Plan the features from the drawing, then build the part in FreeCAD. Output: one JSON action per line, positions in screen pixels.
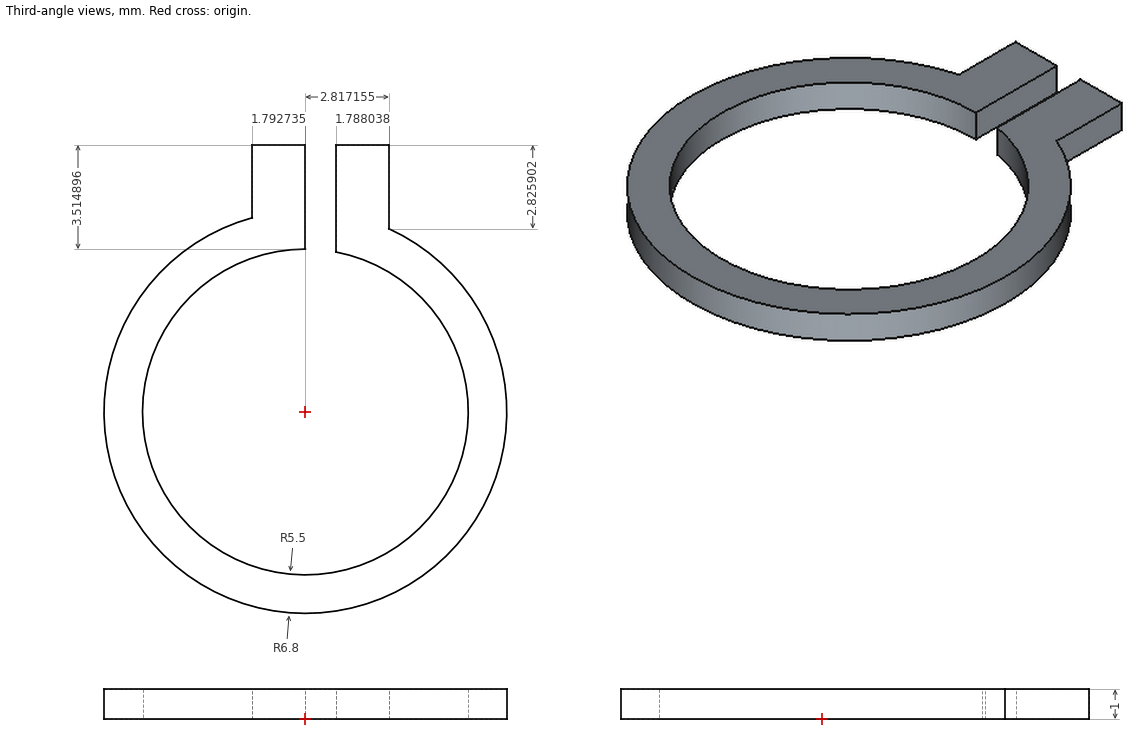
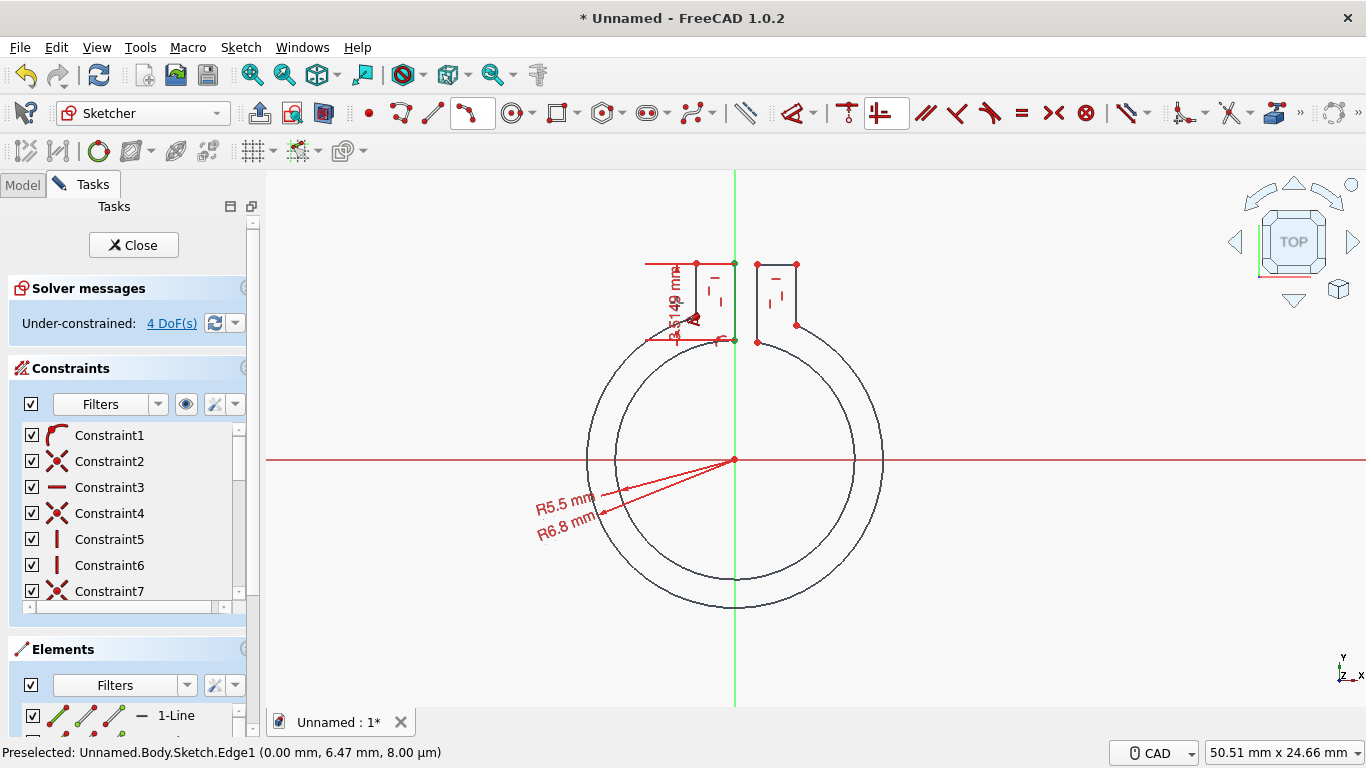
{"action": "left_click", "coordinate": [723, 264]}
{"action": "left_click", "coordinate": [715, 230]}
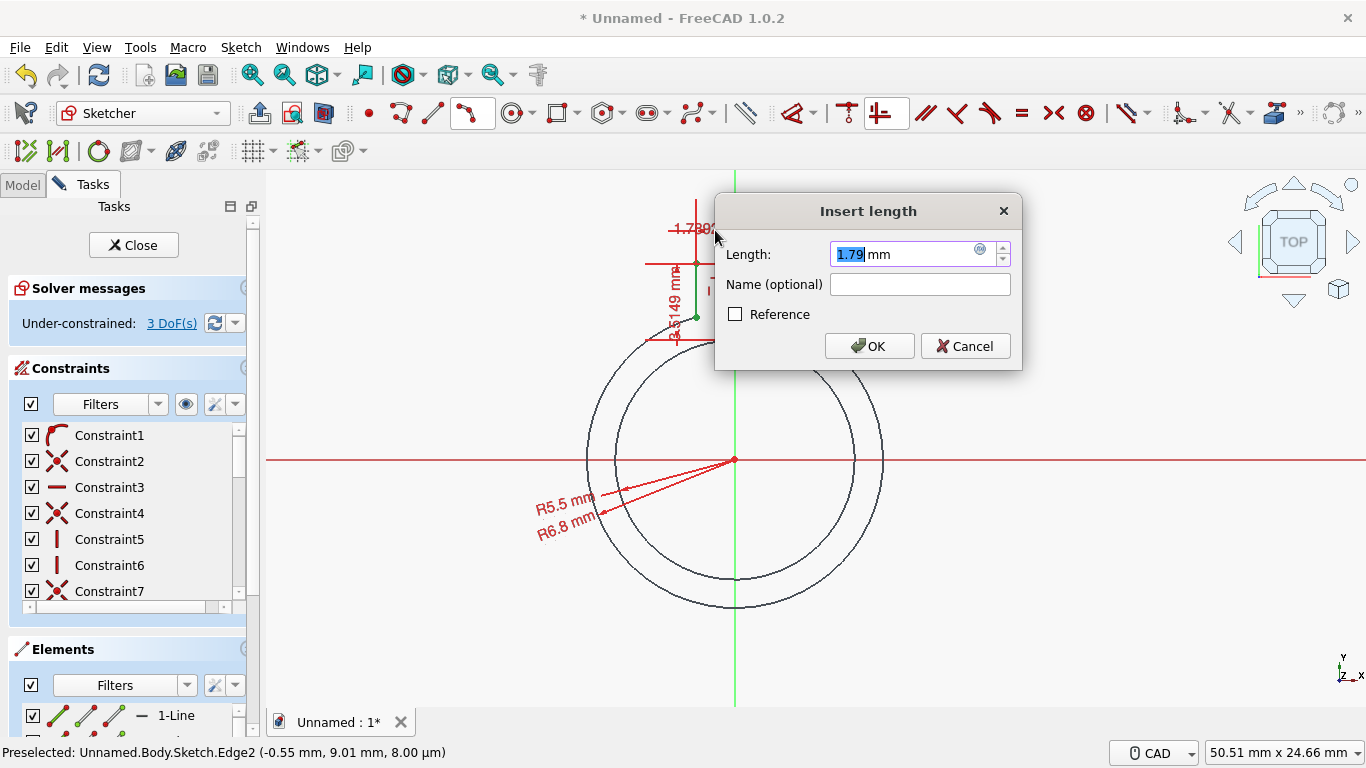
{"action": "type", "text": "1.792735"}
{"action": "key", "text": "Return"}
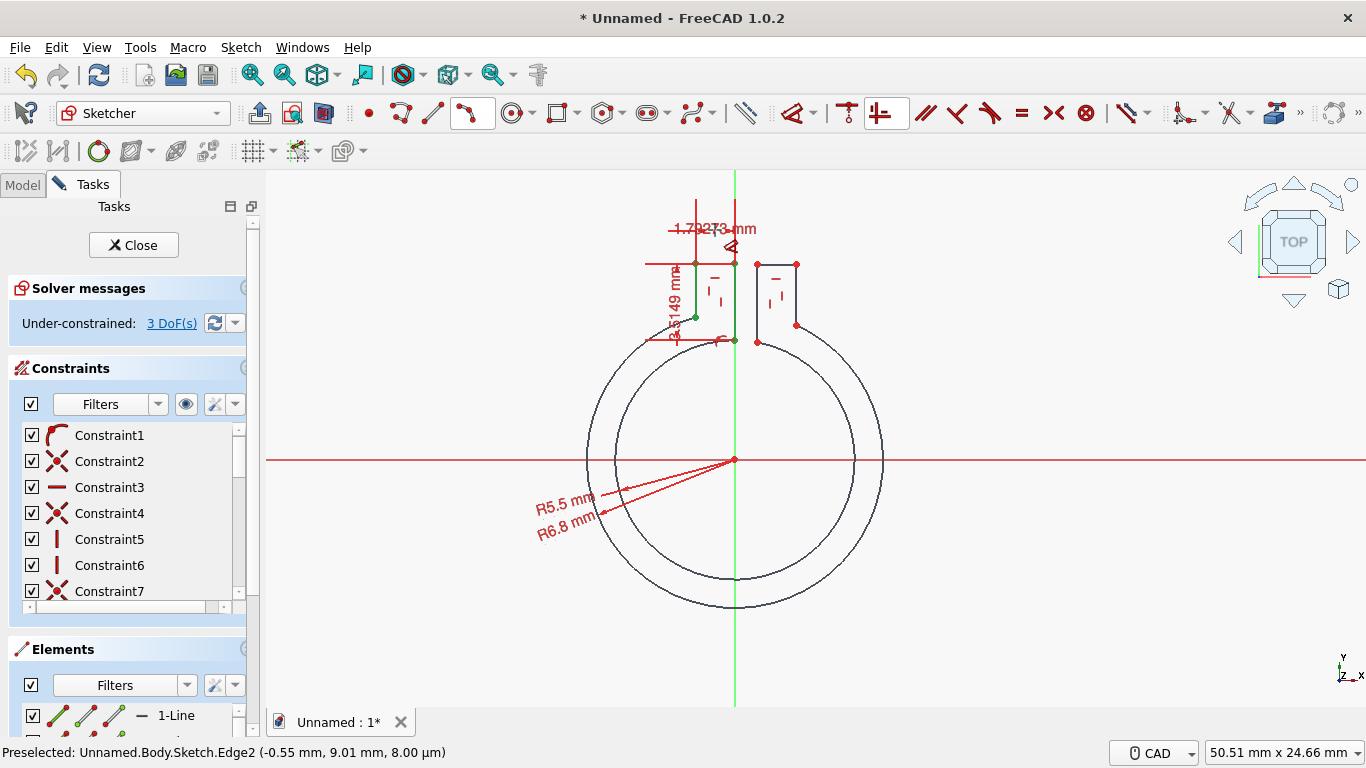
{"action": "left_click", "coordinate": [796, 307]}
{"action": "left_click", "coordinate": [830, 295]}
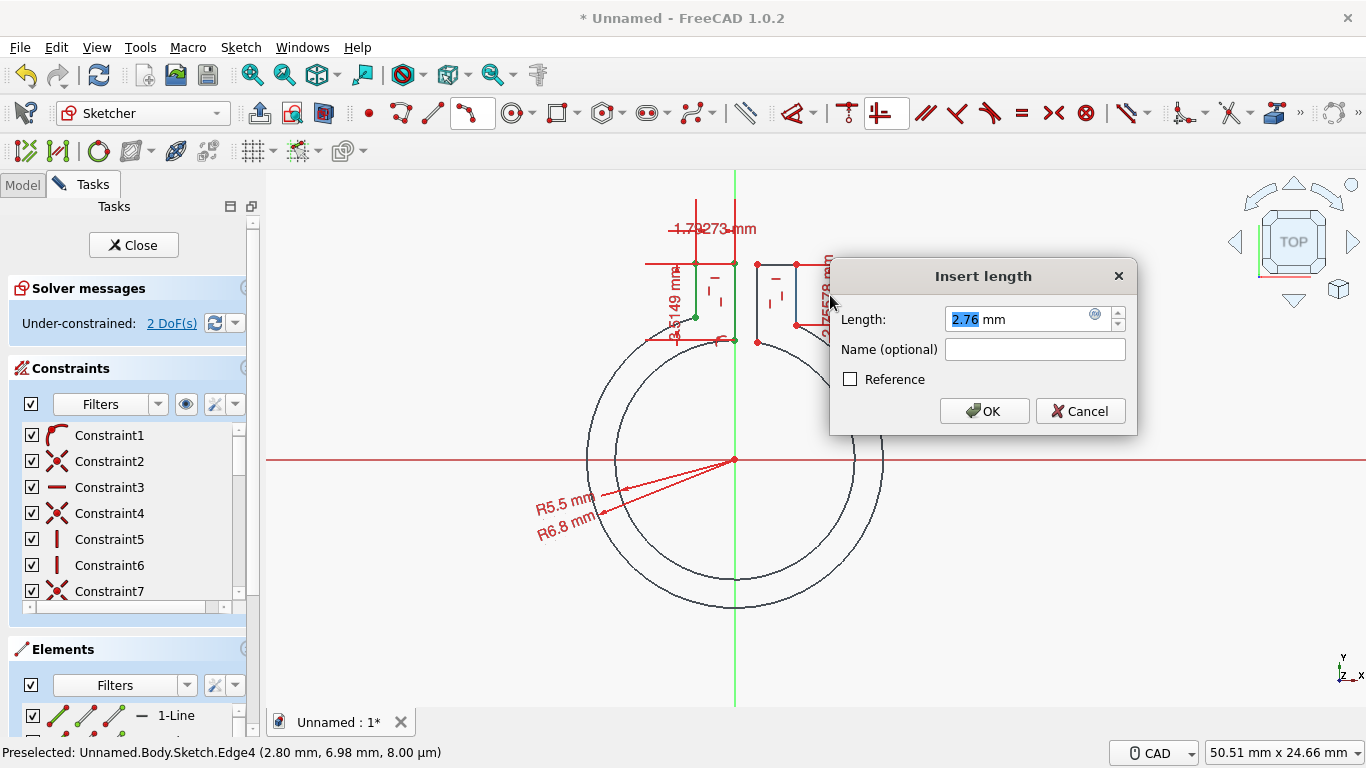
{"action": "type", "text": "2.825902"}
{"action": "key", "text": "Return"}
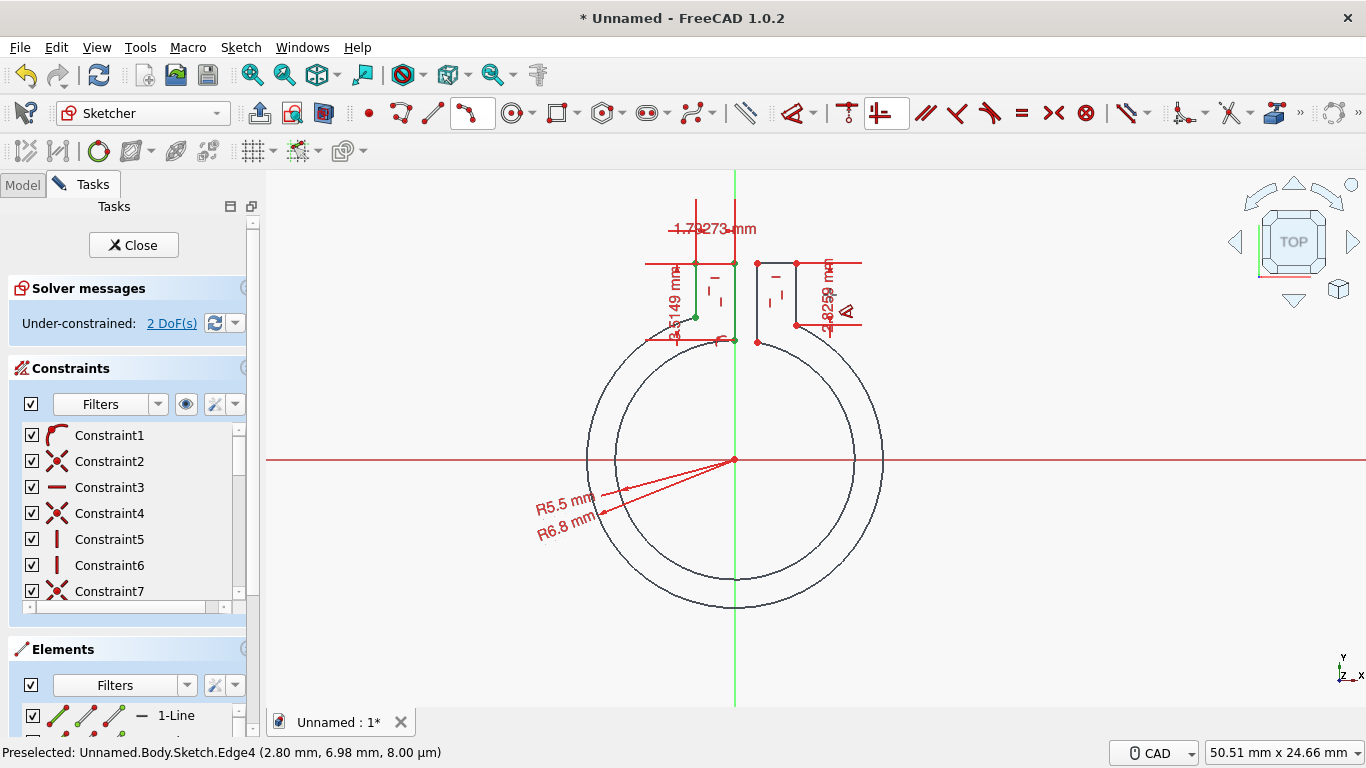
{"action": "left_click", "coordinate": [784, 263]}
{"action": "left_click", "coordinate": [790, 229]}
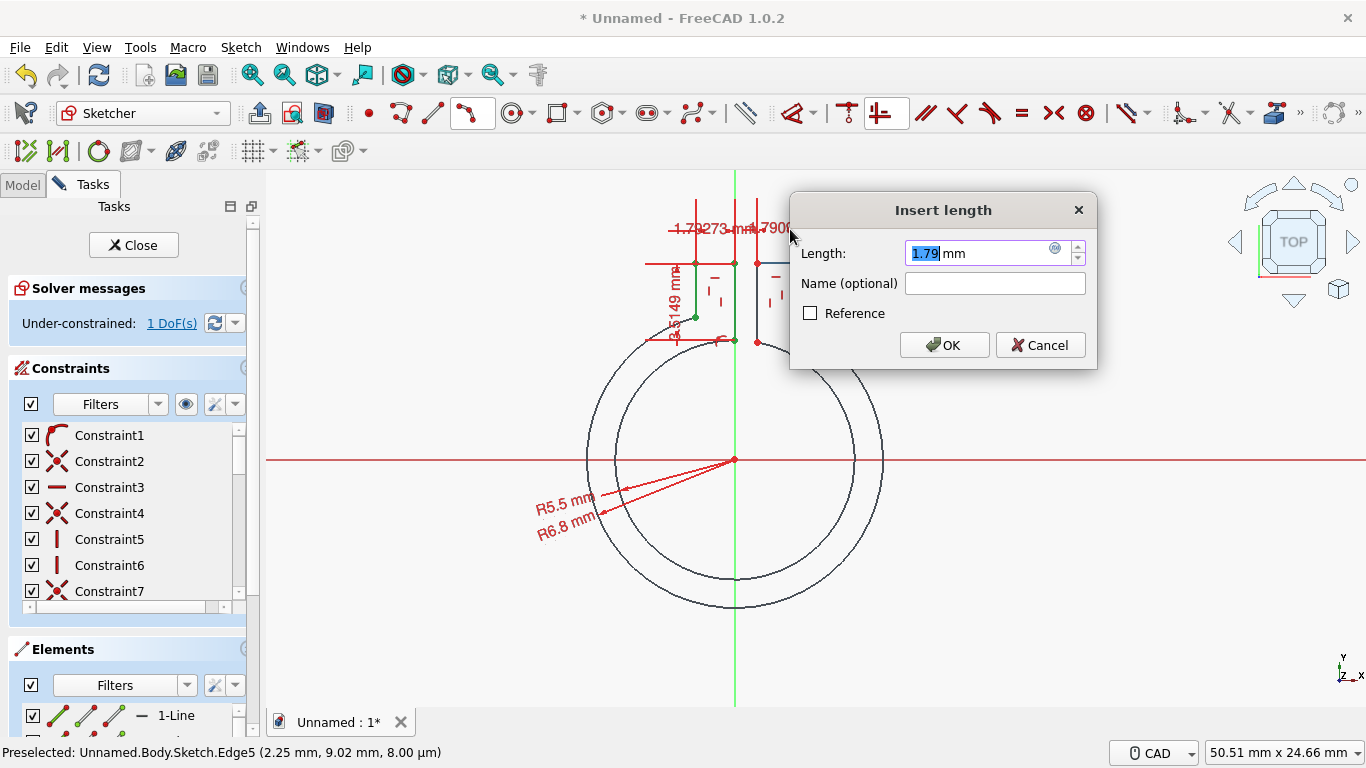
{"action": "type", "text": "1.788038"}
{"action": "key", "text": "Return"}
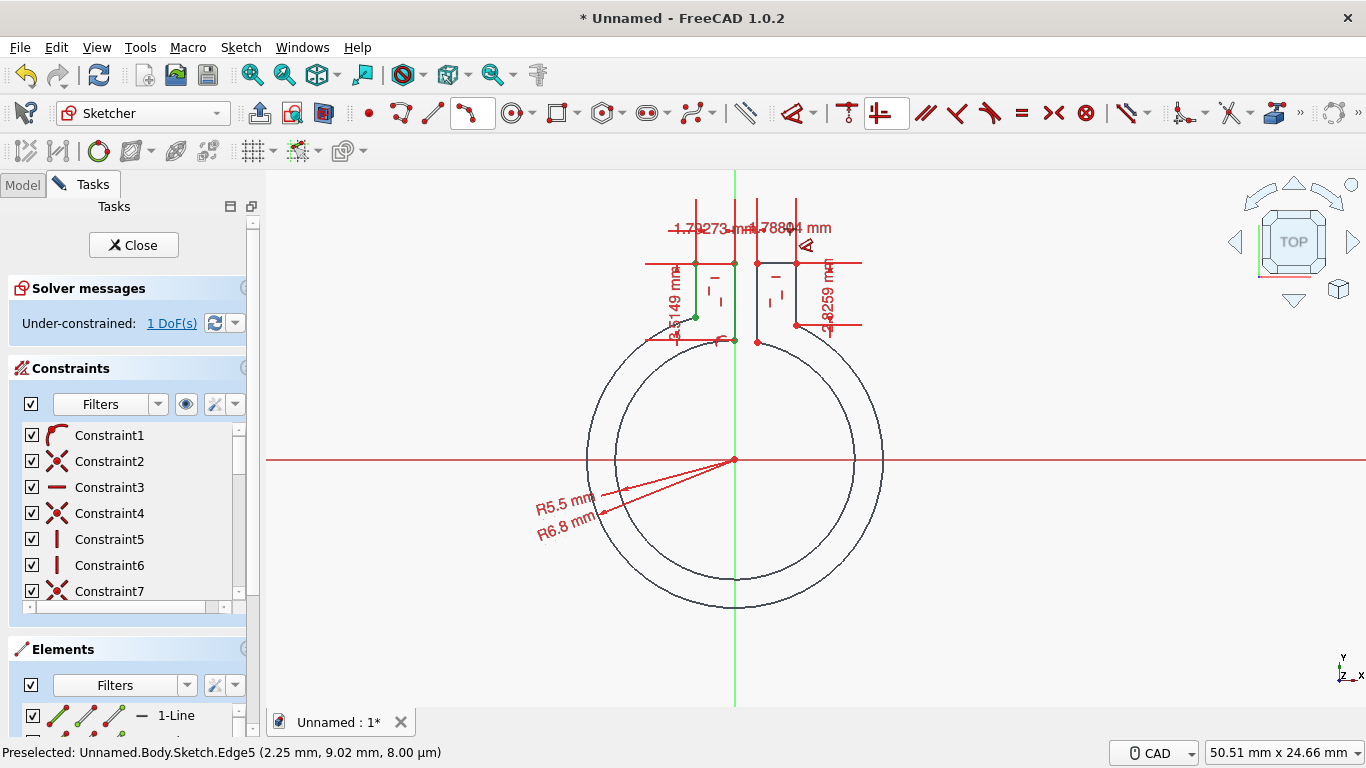
{"action": "left_click", "coordinate": [796, 325]}
{"action": "left_click", "coordinate": [765, 494]}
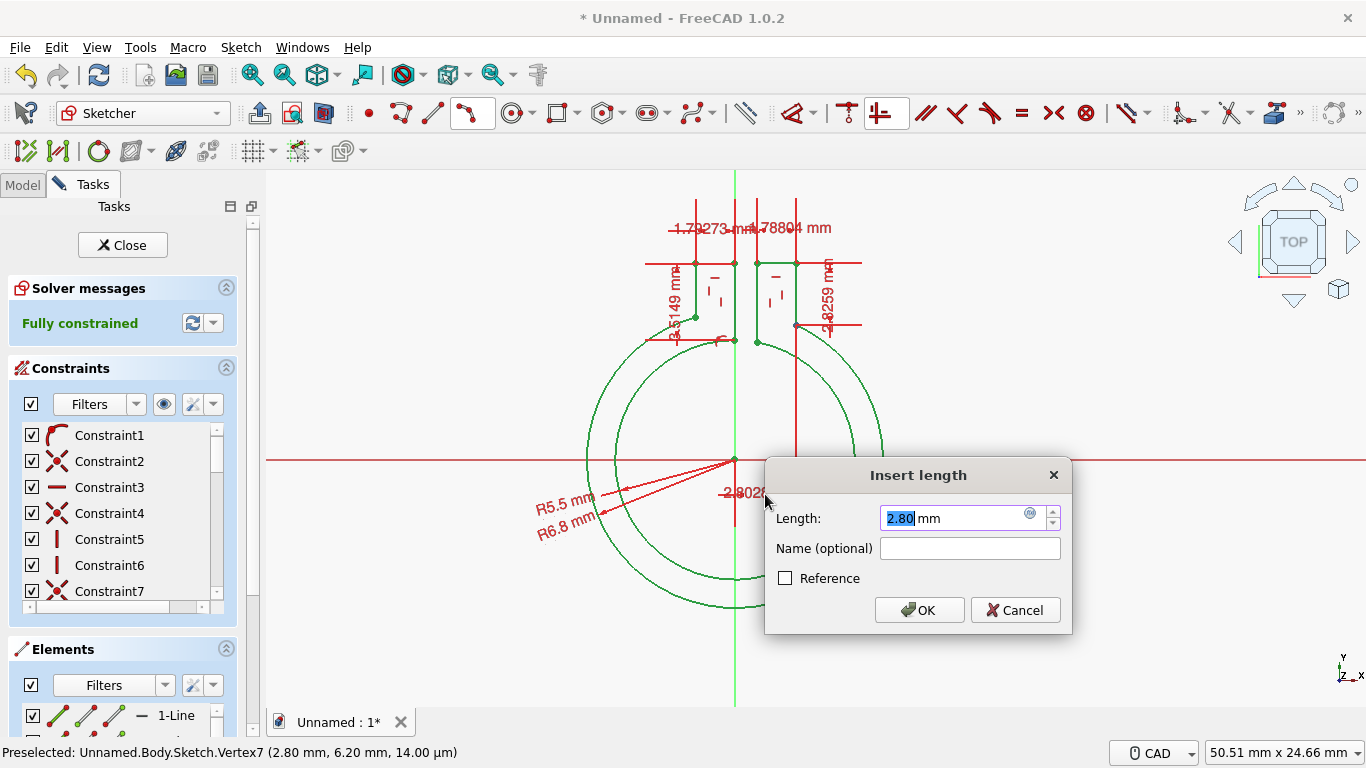
{"action": "type", "text": "2.817155"}
{"action": "key", "text": "Return"}
{"action": "key", "text": "Escape"}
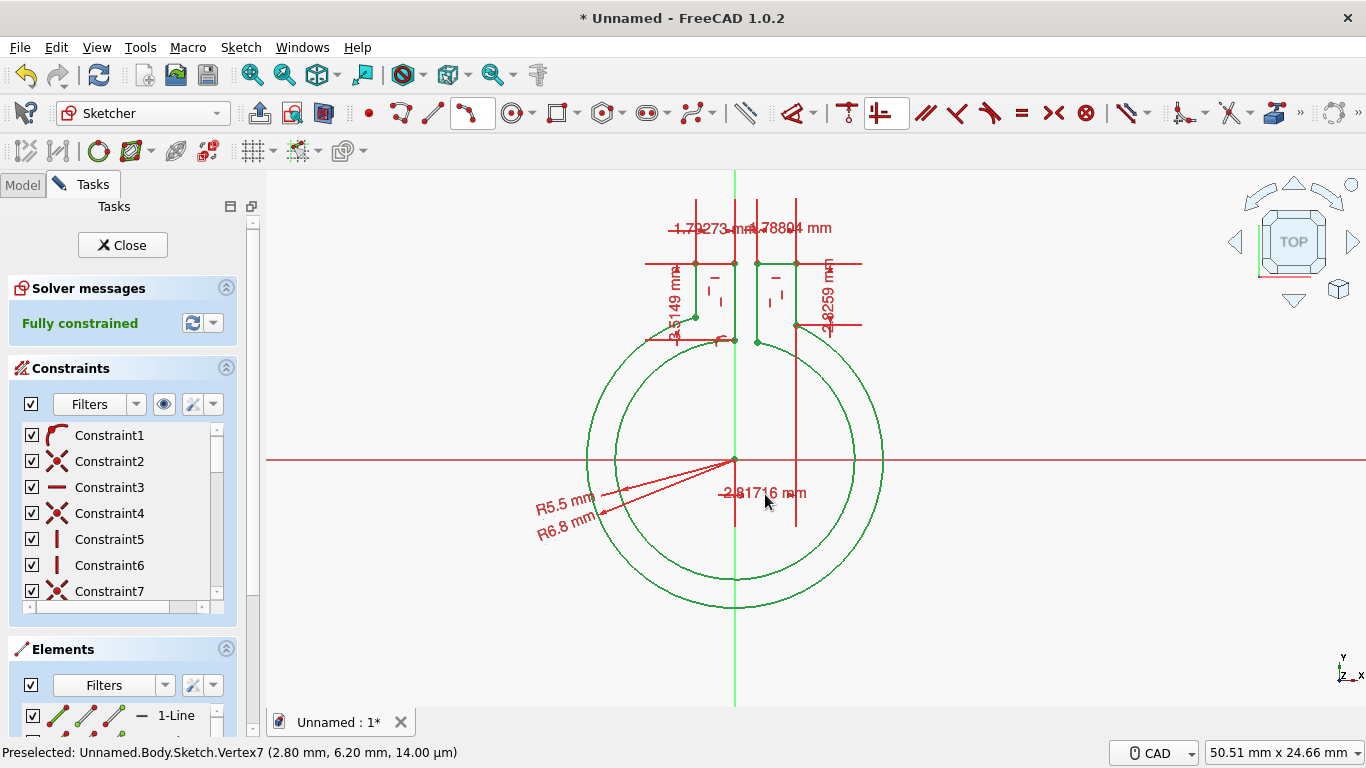
{"action": "left_click", "coordinate": [123, 245]}